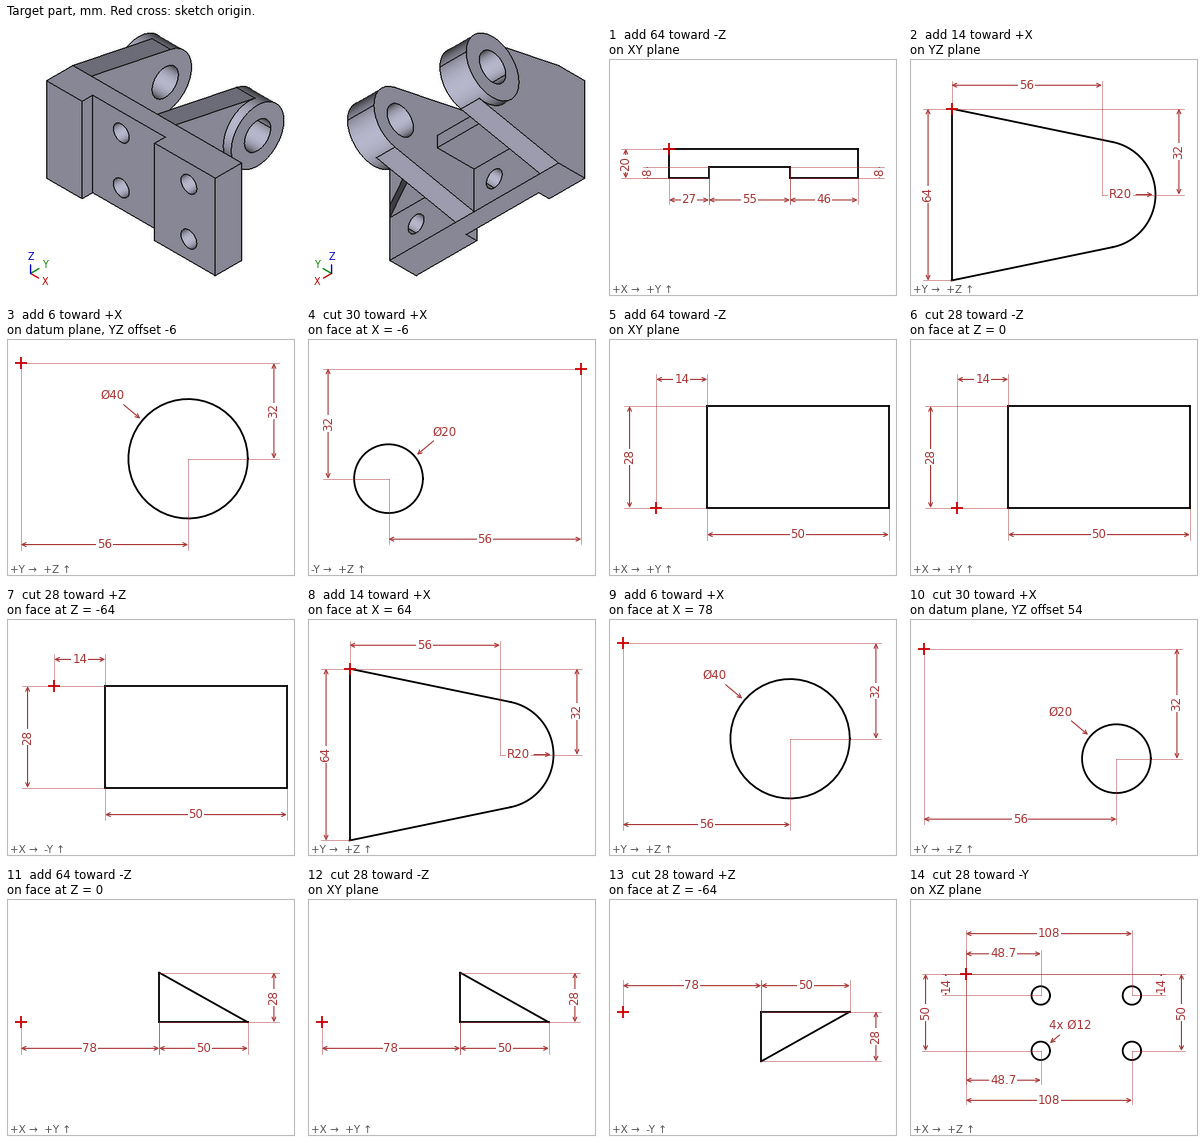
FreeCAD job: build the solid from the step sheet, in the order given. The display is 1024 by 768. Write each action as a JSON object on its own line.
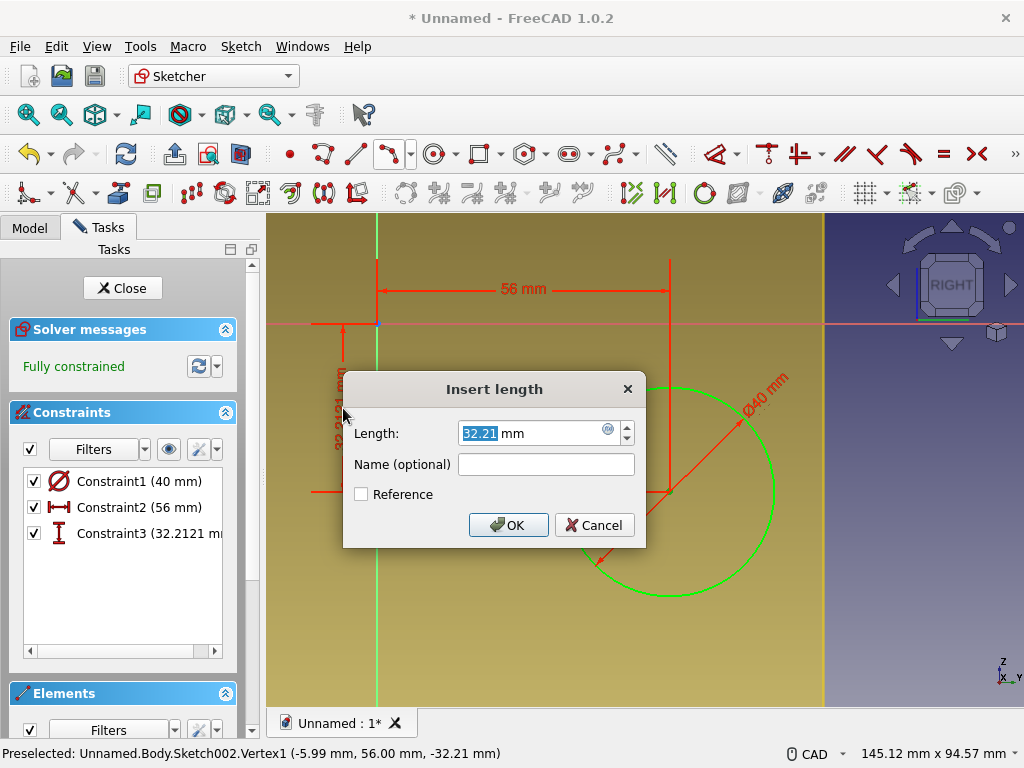
{"action": "type", "text": "32"}
{"action": "key", "text": "Return"}
{"action": "key", "text": "Escape"}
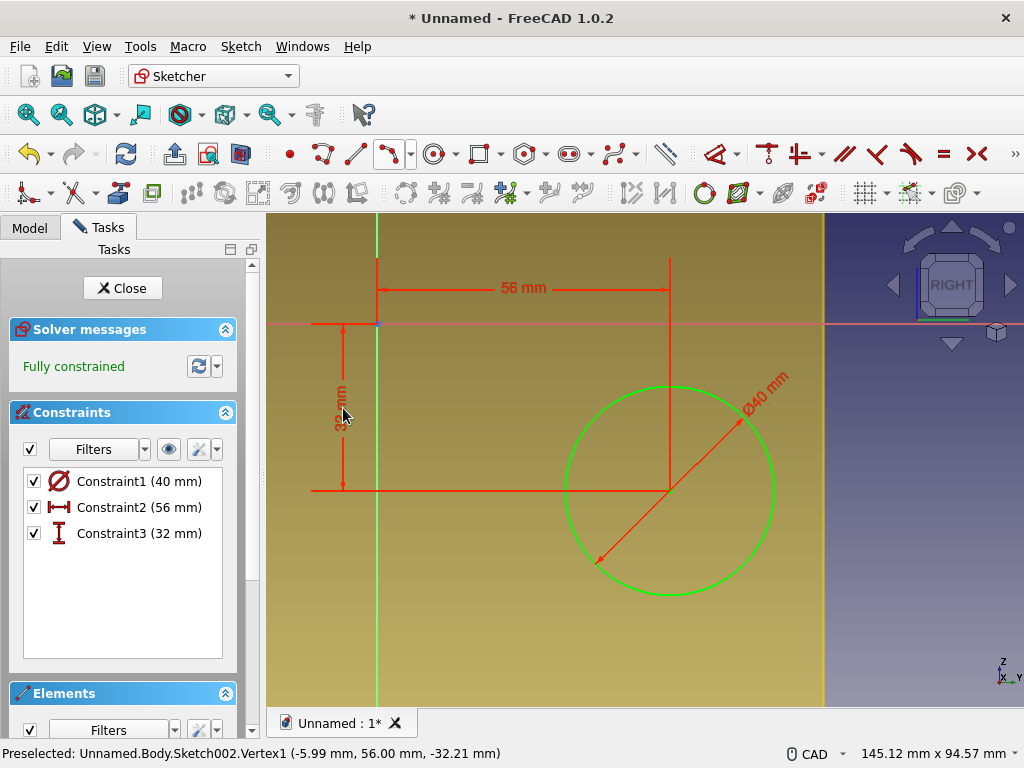
{"action": "left_click", "coordinate": [123, 288]}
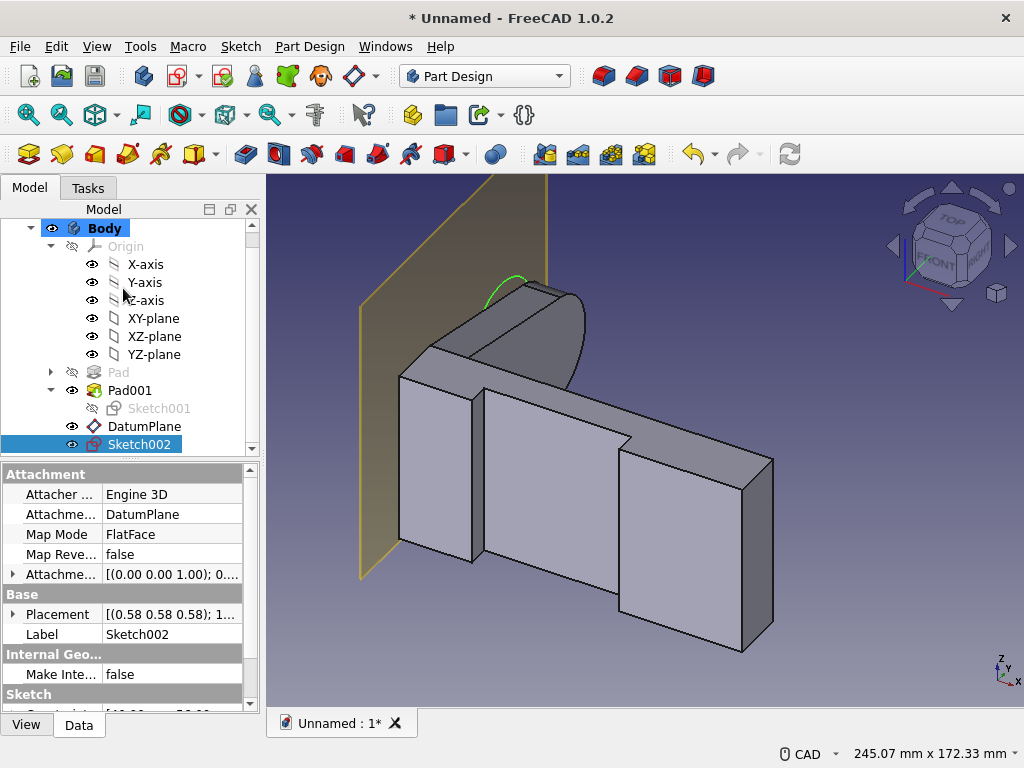
{"action": "left_click", "coordinate": [29, 154]}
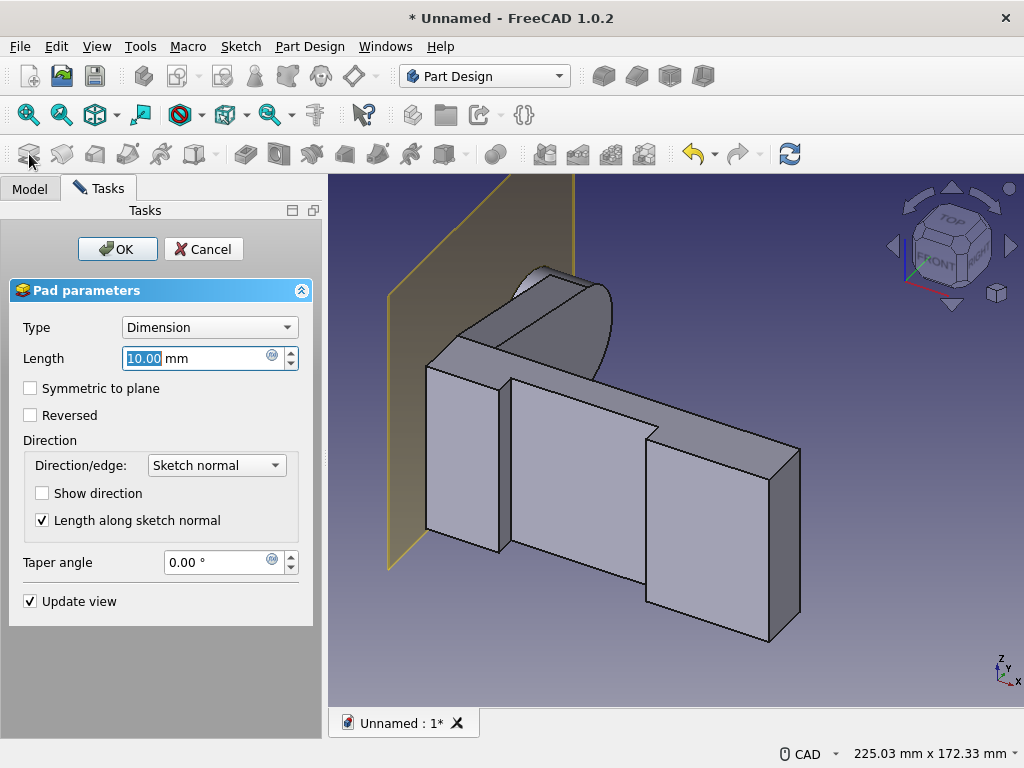
{"action": "type", "text": "6"}
{"action": "key", "text": "Tab"}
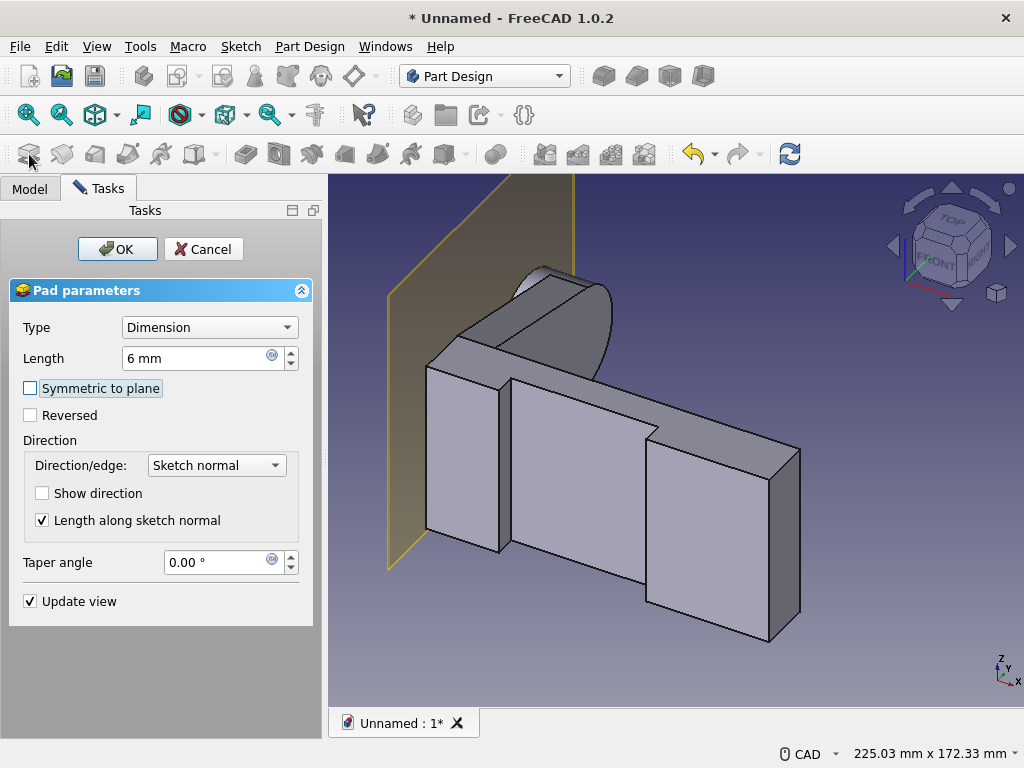
{"action": "left_click", "coordinate": [118, 249]}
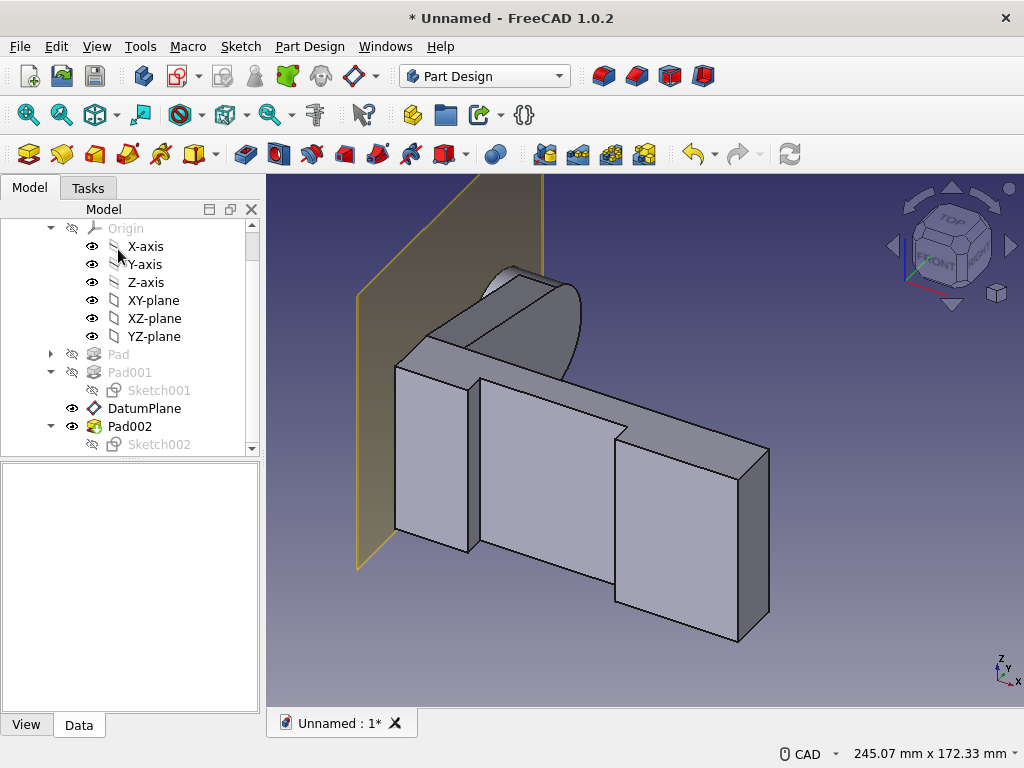
{"action": "left_click", "coordinate": [117, 408]}
{"action": "key", "text": "space"}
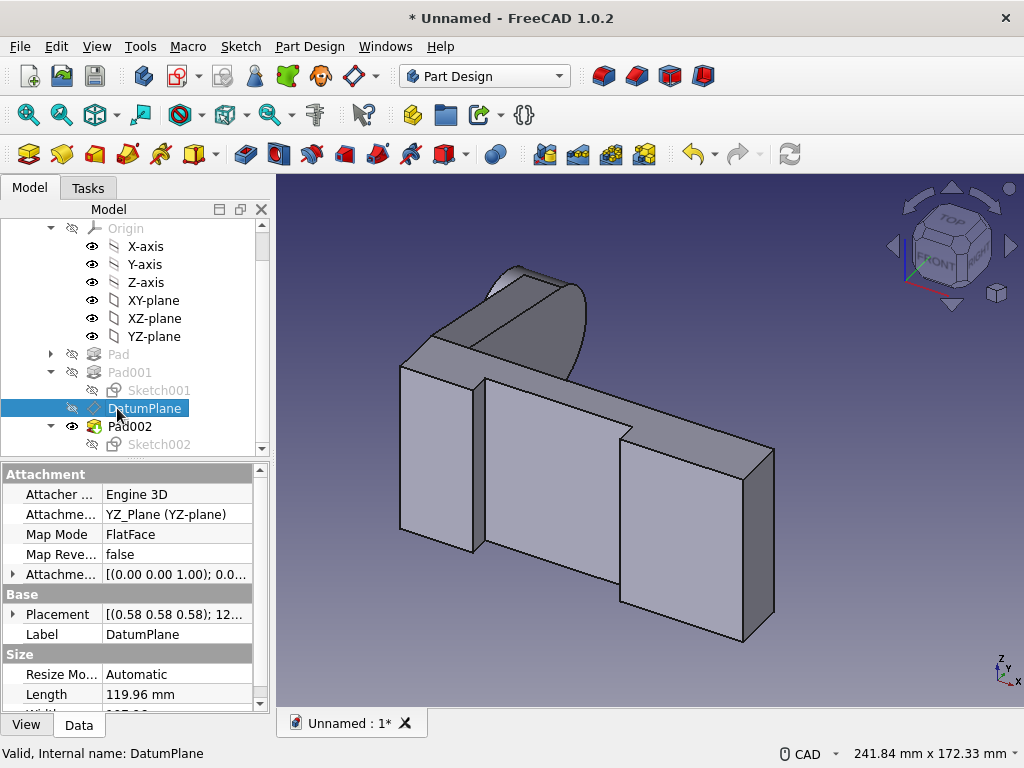
{"action": "key", "text": "6"}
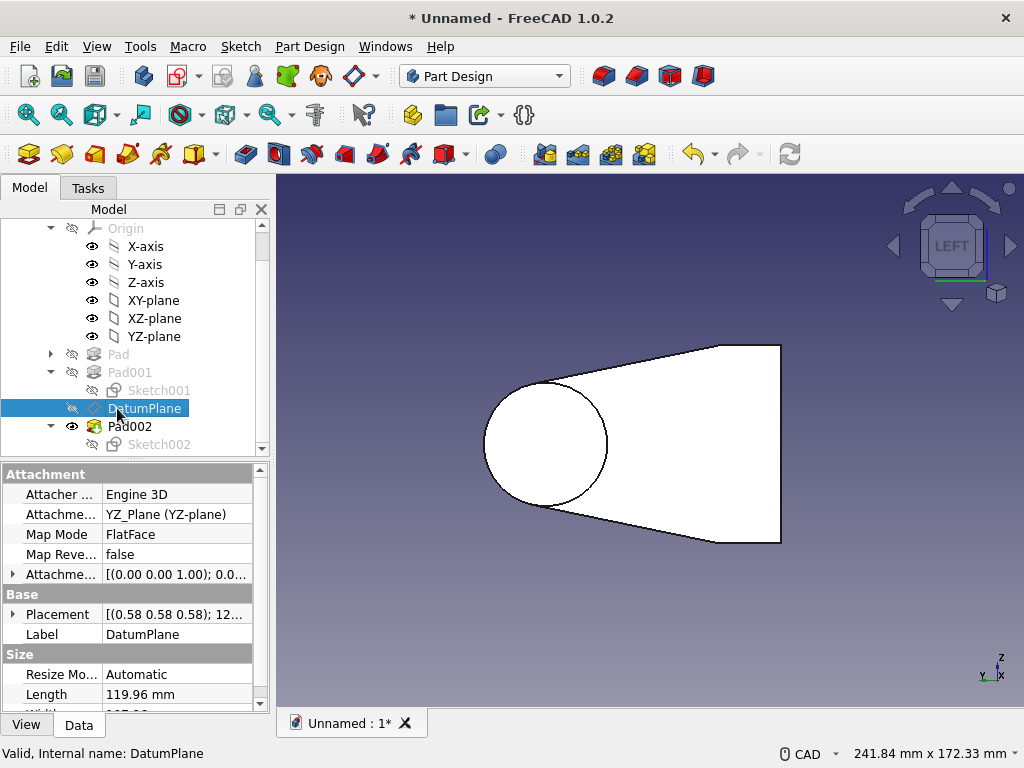
{"action": "left_click", "coordinate": [29, 116]}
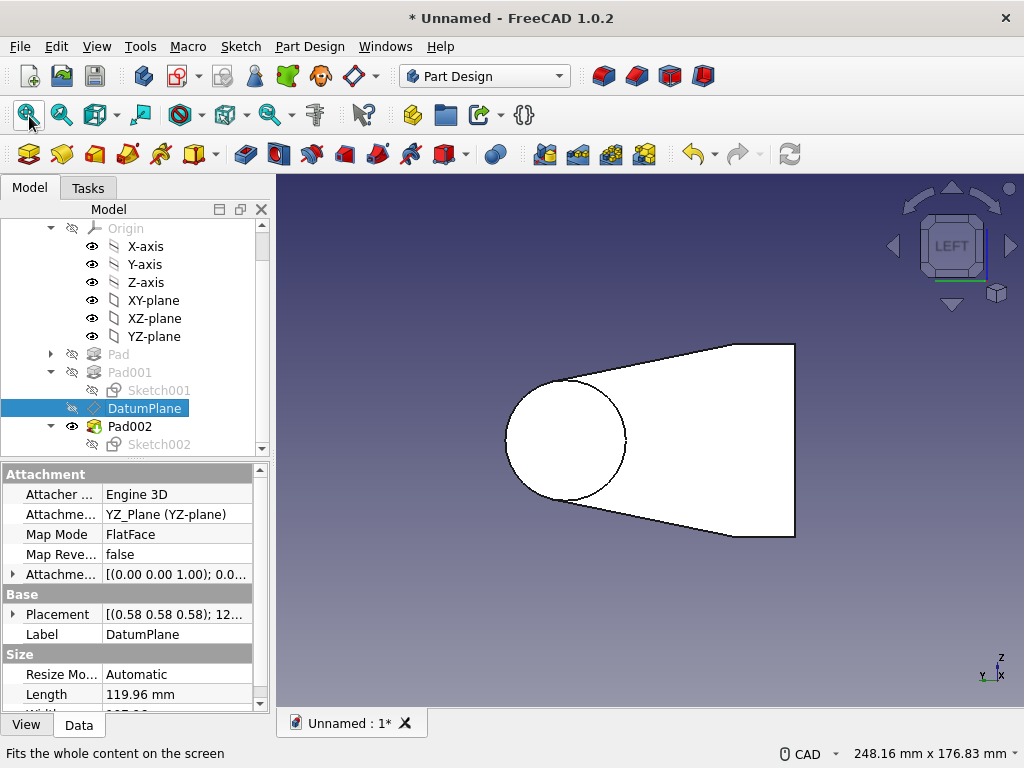
{"action": "left_click", "coordinate": [566, 439]}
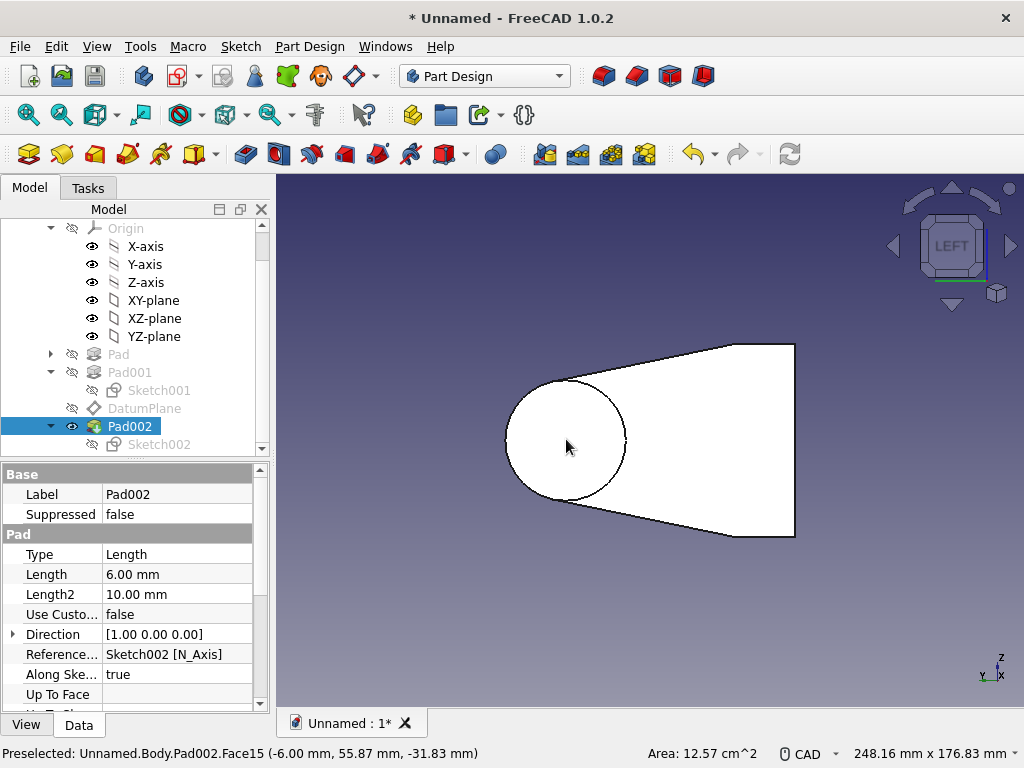
{"action": "left_click", "coordinate": [176, 76]}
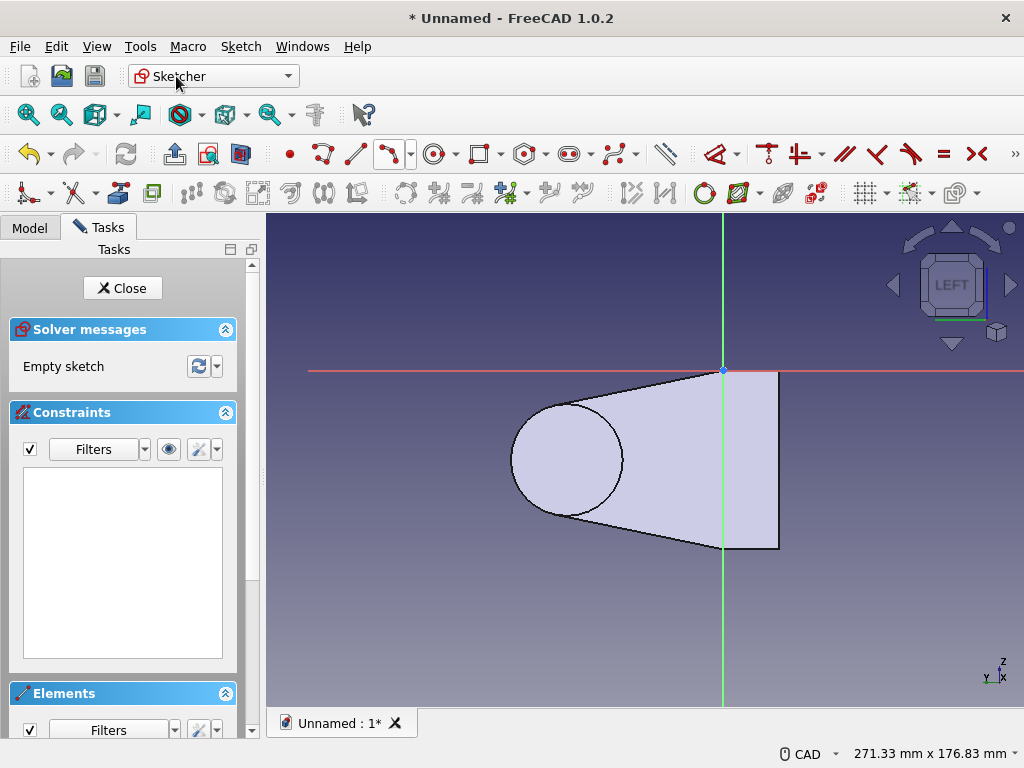
{"action": "scroll", "coordinate": [565, 460], "scroll_direction": "up", "scroll_amount": 9}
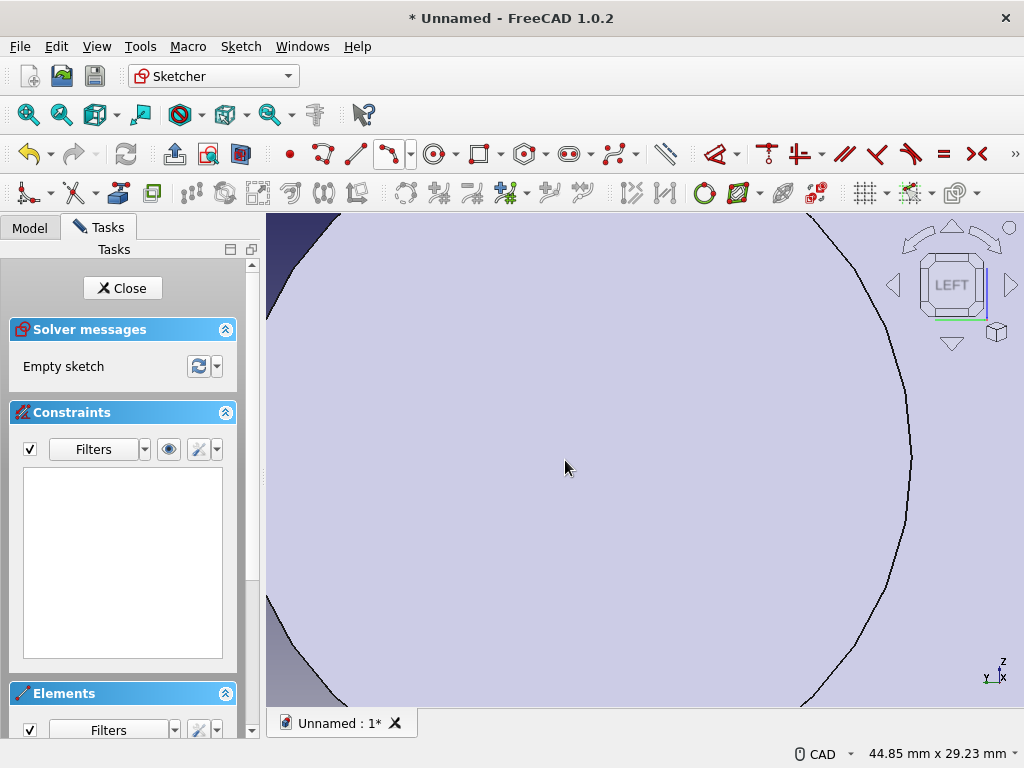
{"action": "left_click", "coordinate": [434, 154]}